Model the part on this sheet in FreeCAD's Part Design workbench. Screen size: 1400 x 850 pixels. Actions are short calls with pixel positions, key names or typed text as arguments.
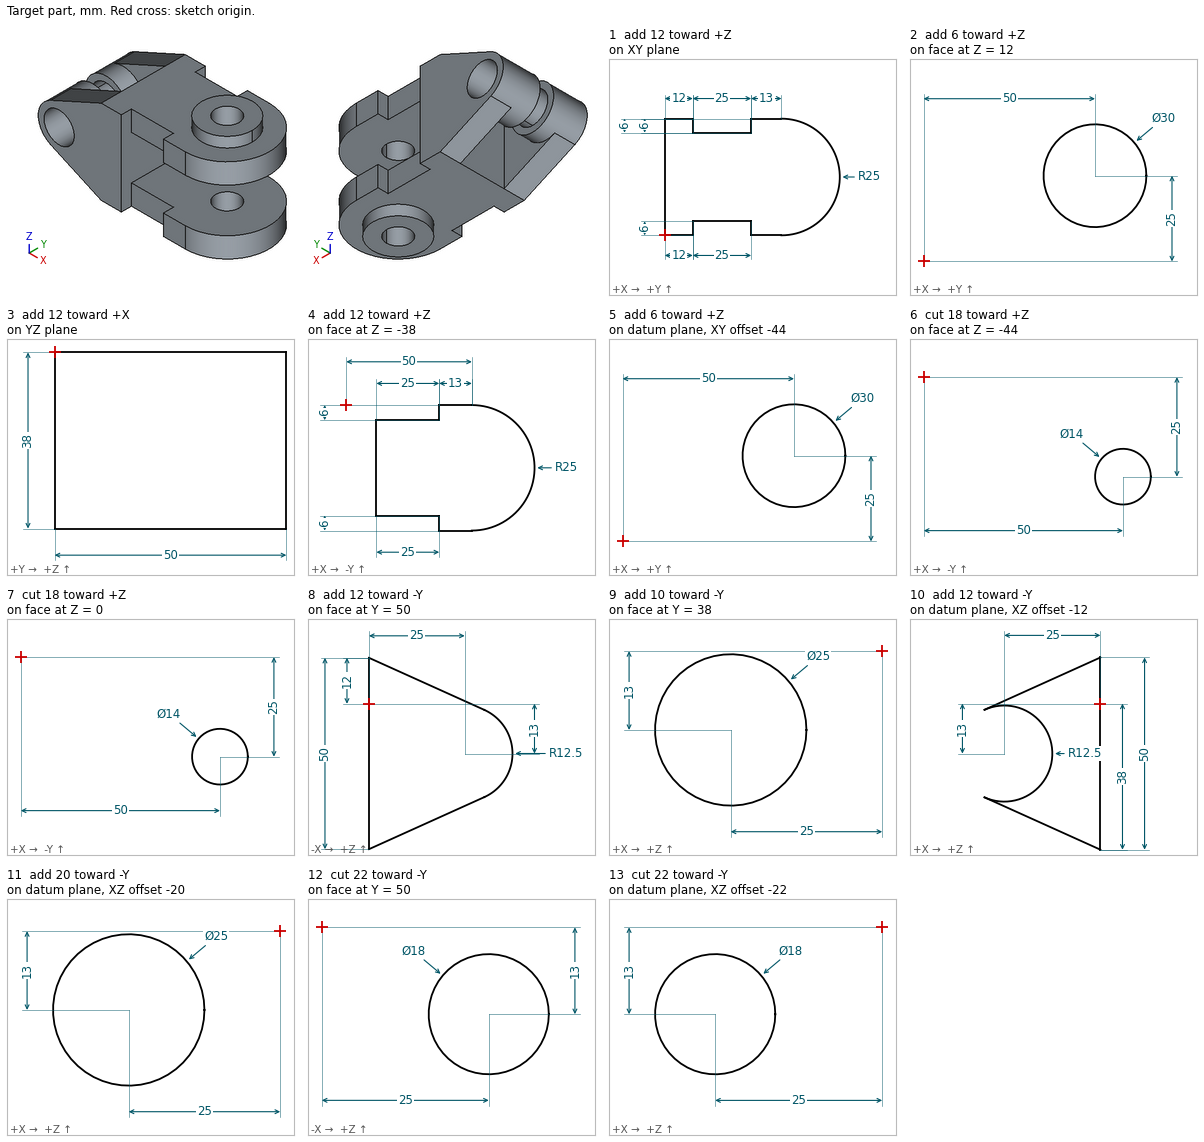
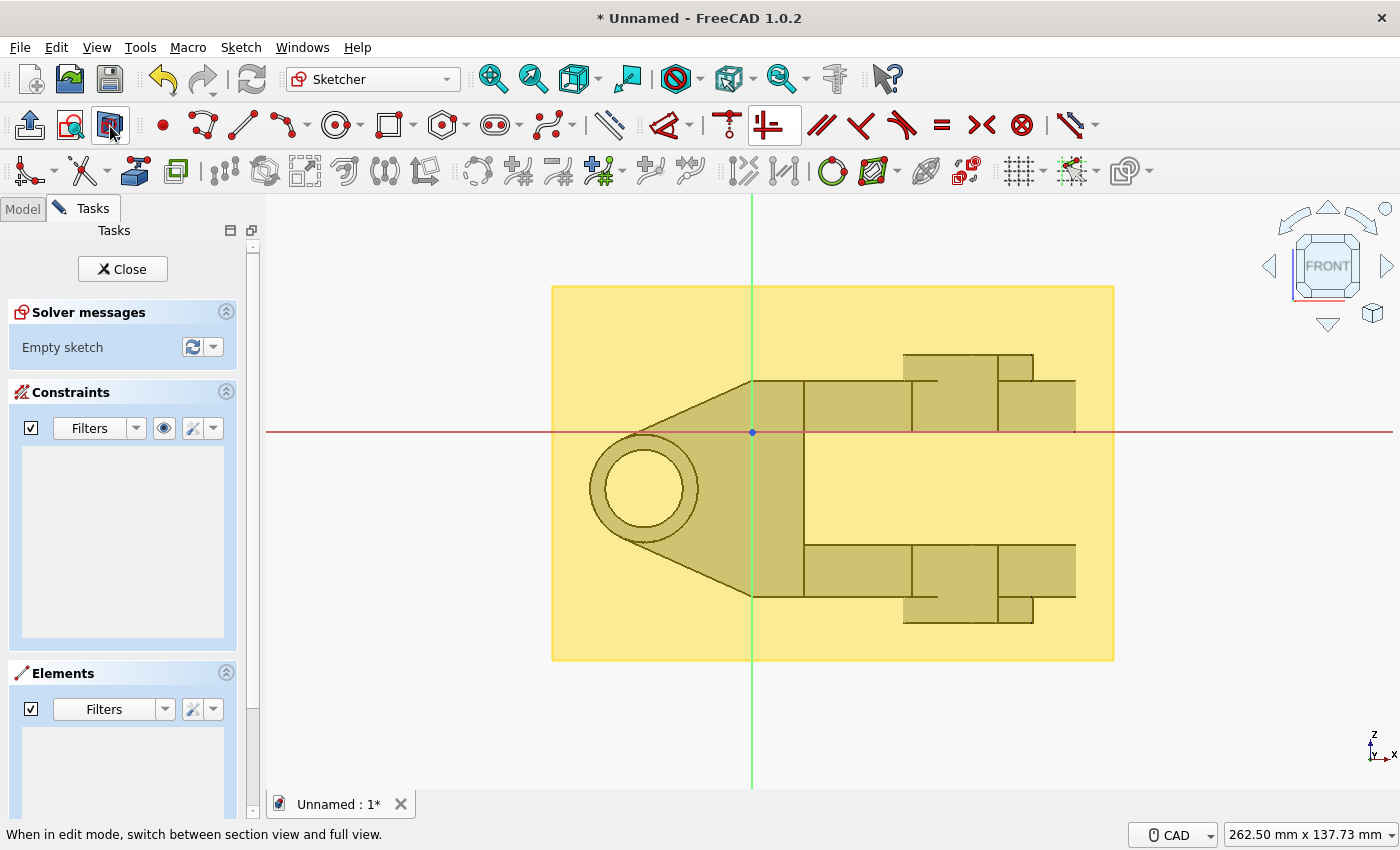
scroll(650, 476, up, 7)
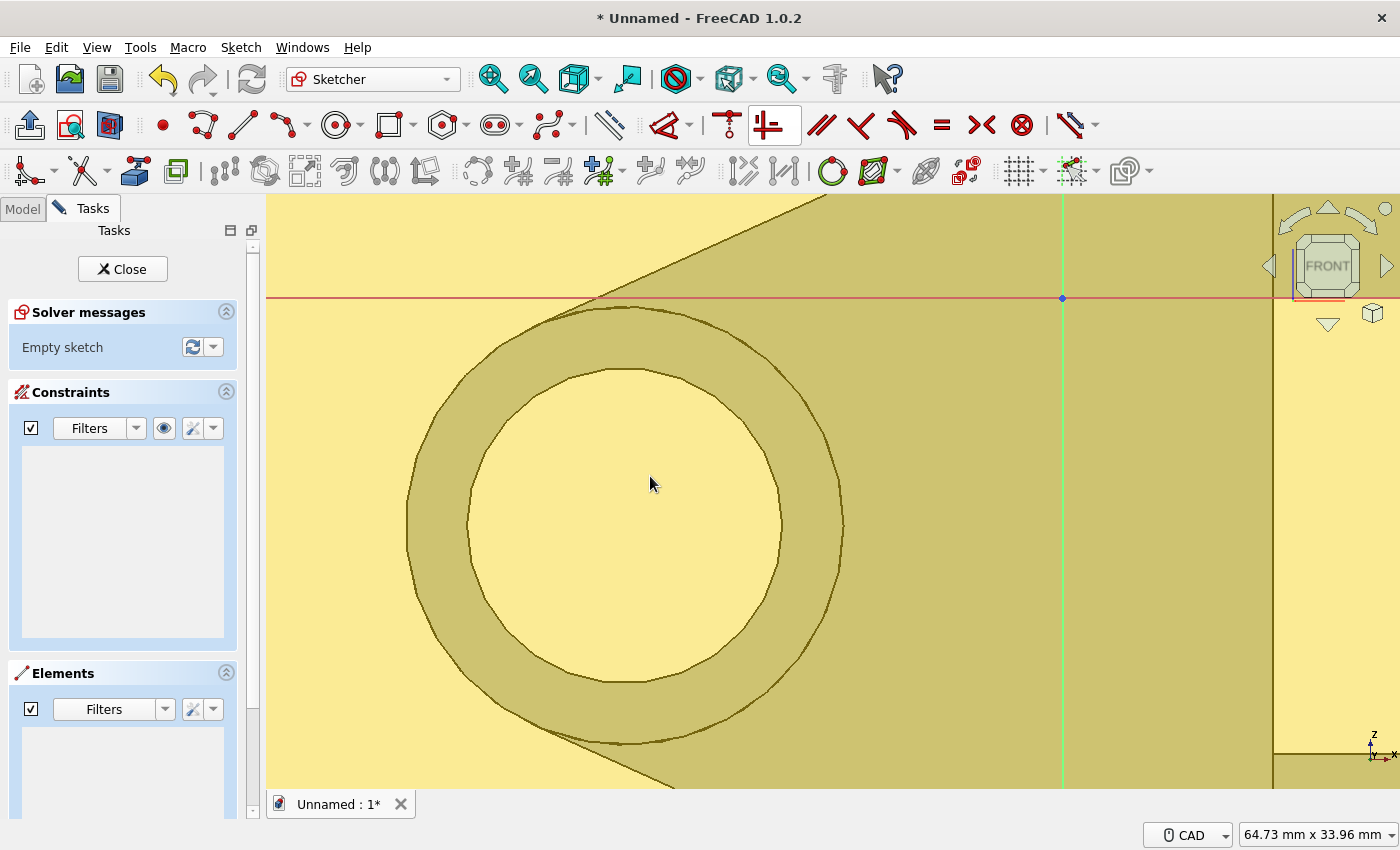
click(336, 126)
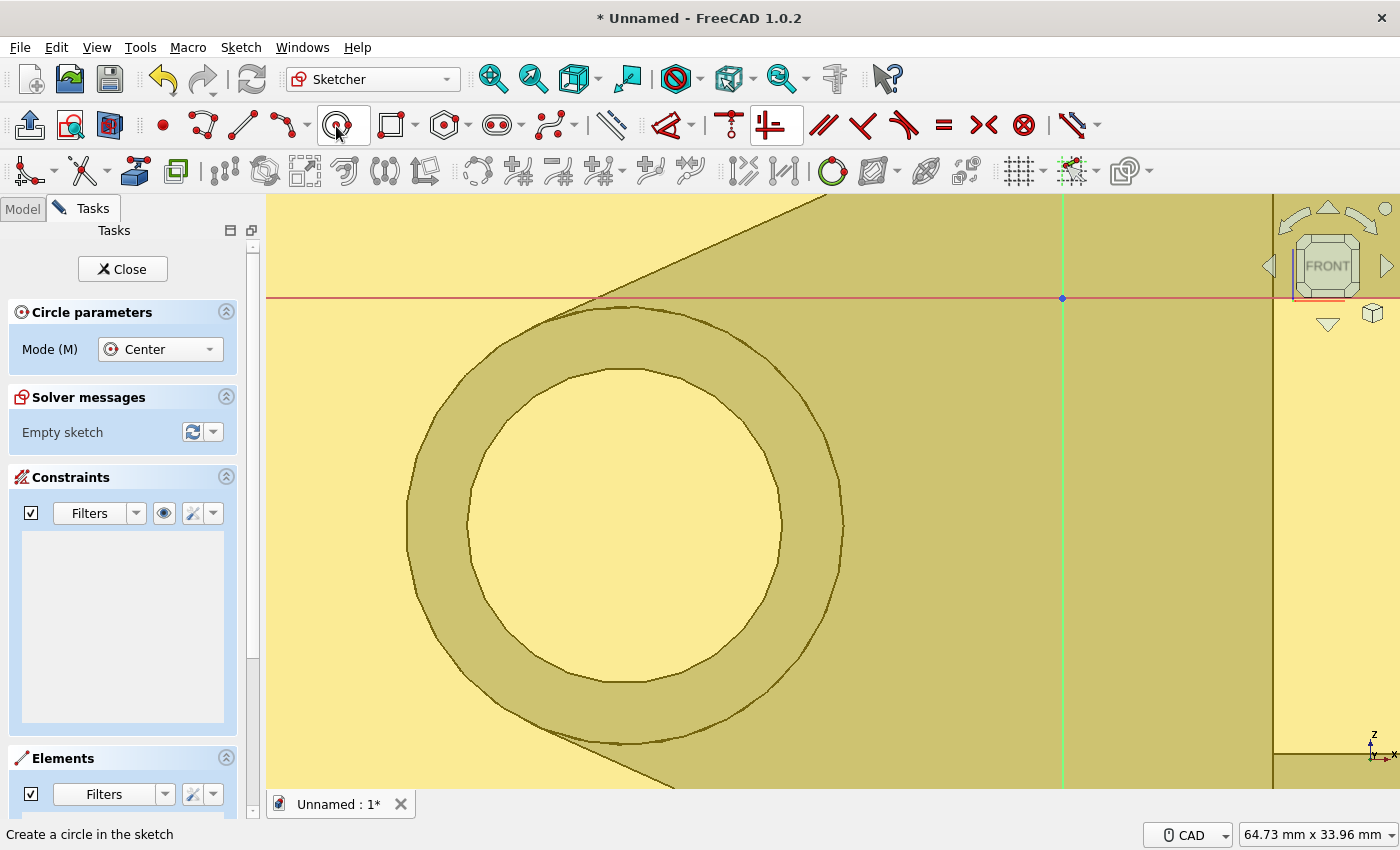
click(625, 526)
click(736, 414)
key(Escape)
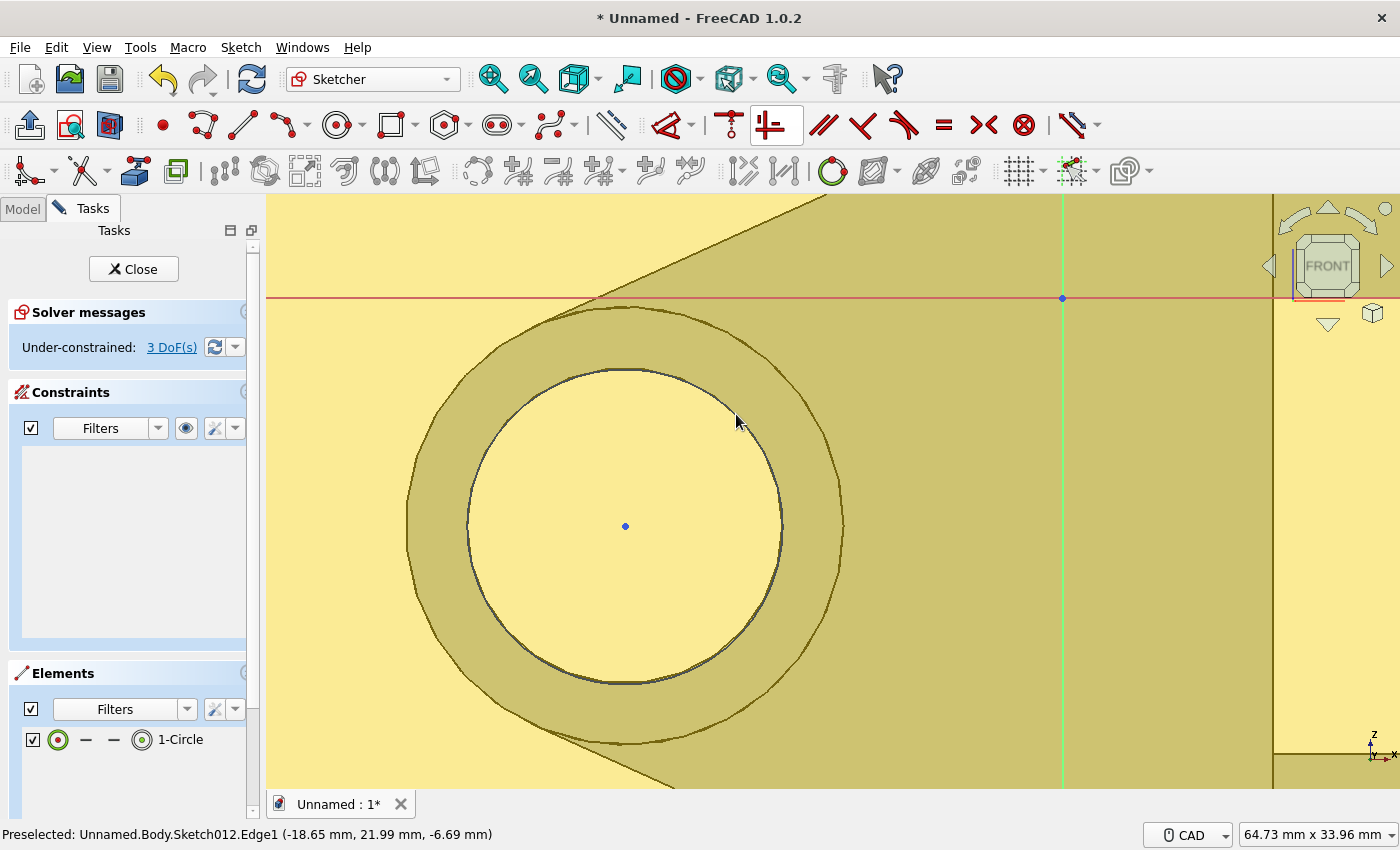
click(666, 126)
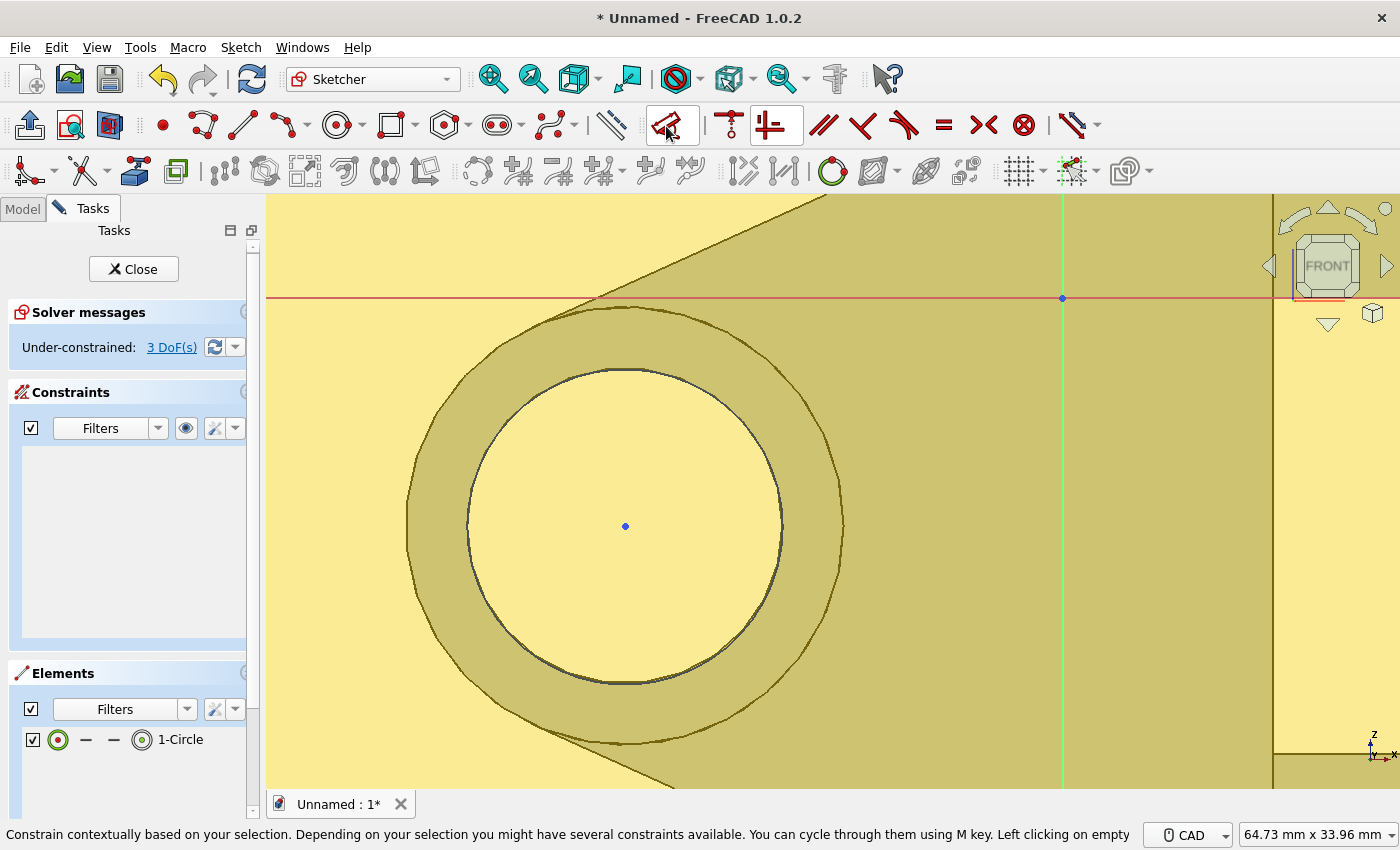
click(736, 415)
click(759, 392)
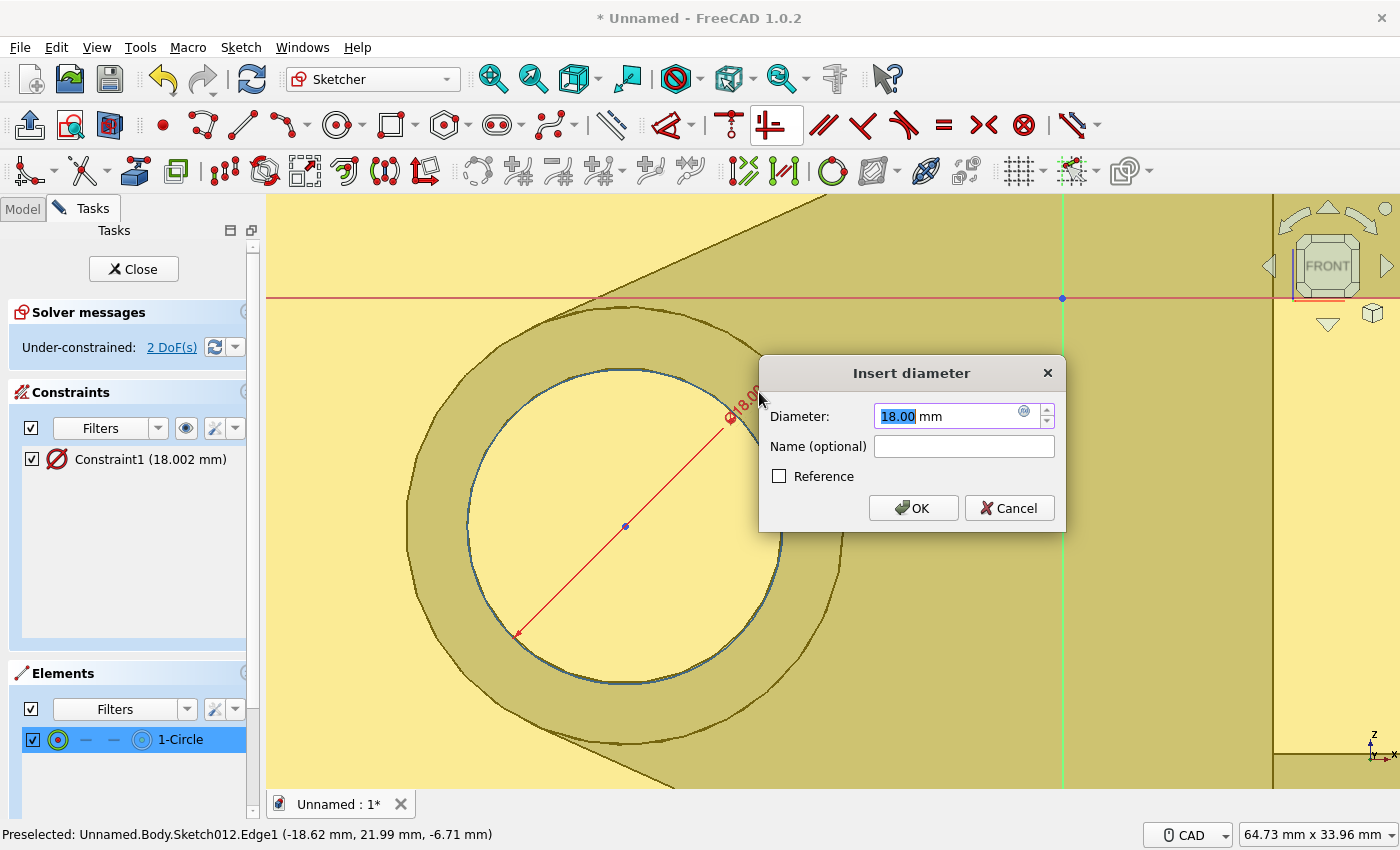
text(18)
key(Return)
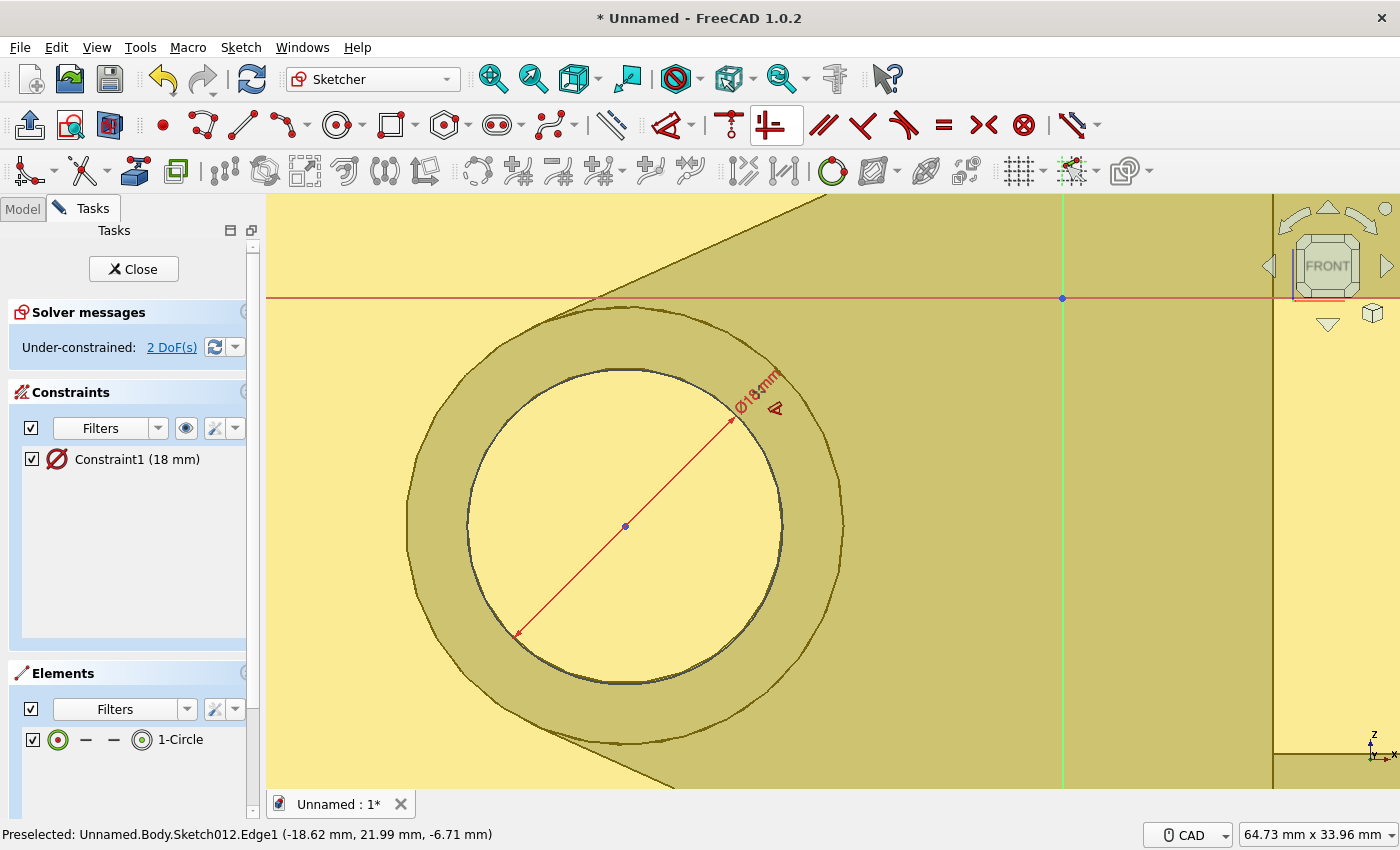
click(625, 527)
click(844, 264)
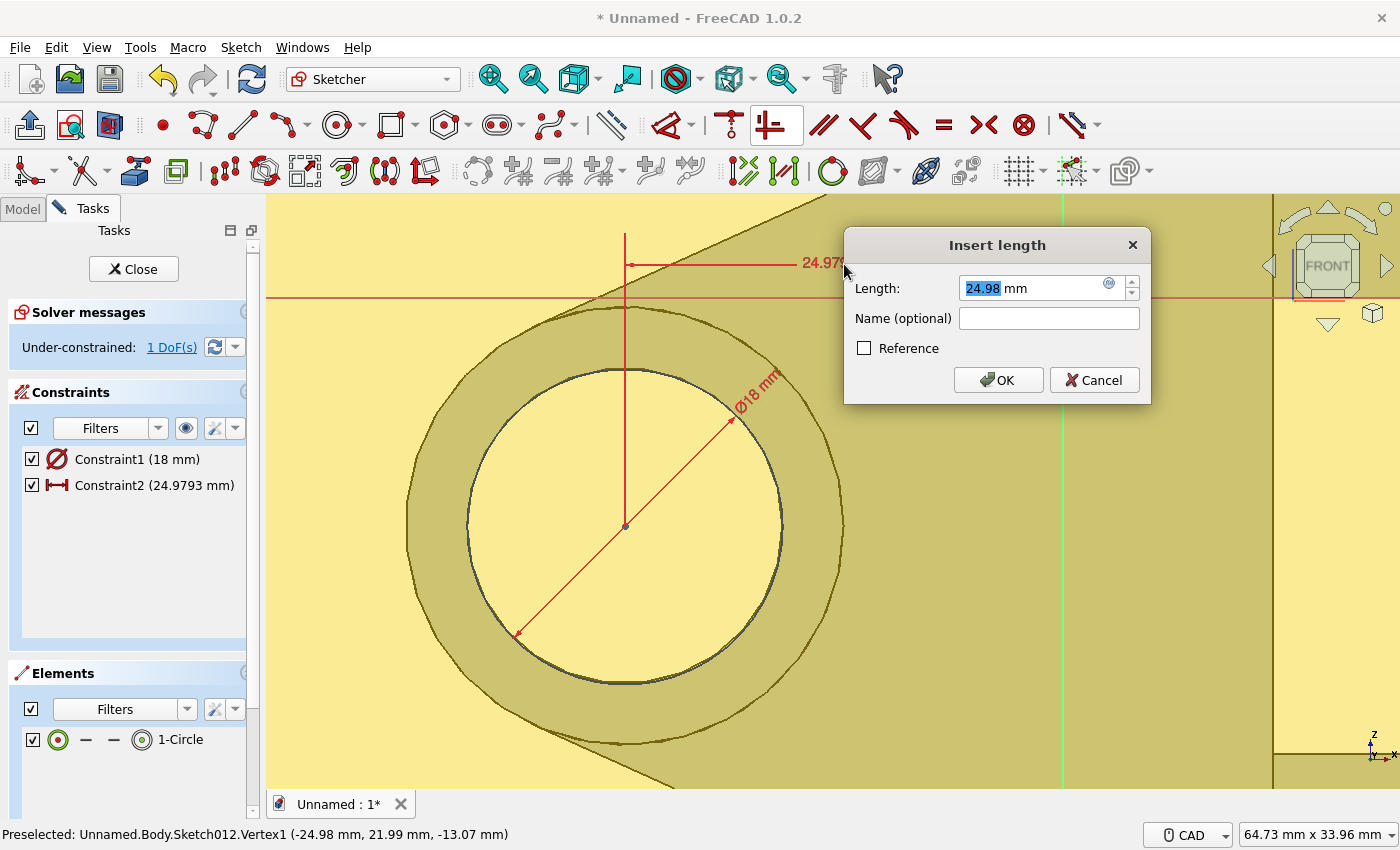
text(25)
key(Return)